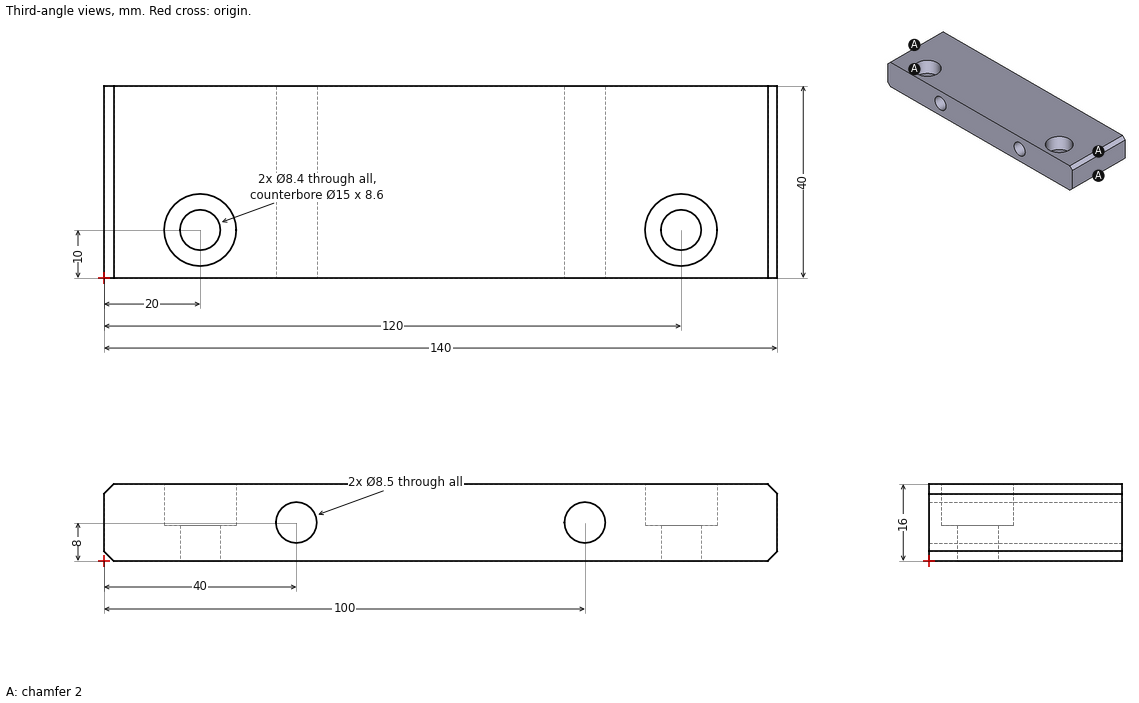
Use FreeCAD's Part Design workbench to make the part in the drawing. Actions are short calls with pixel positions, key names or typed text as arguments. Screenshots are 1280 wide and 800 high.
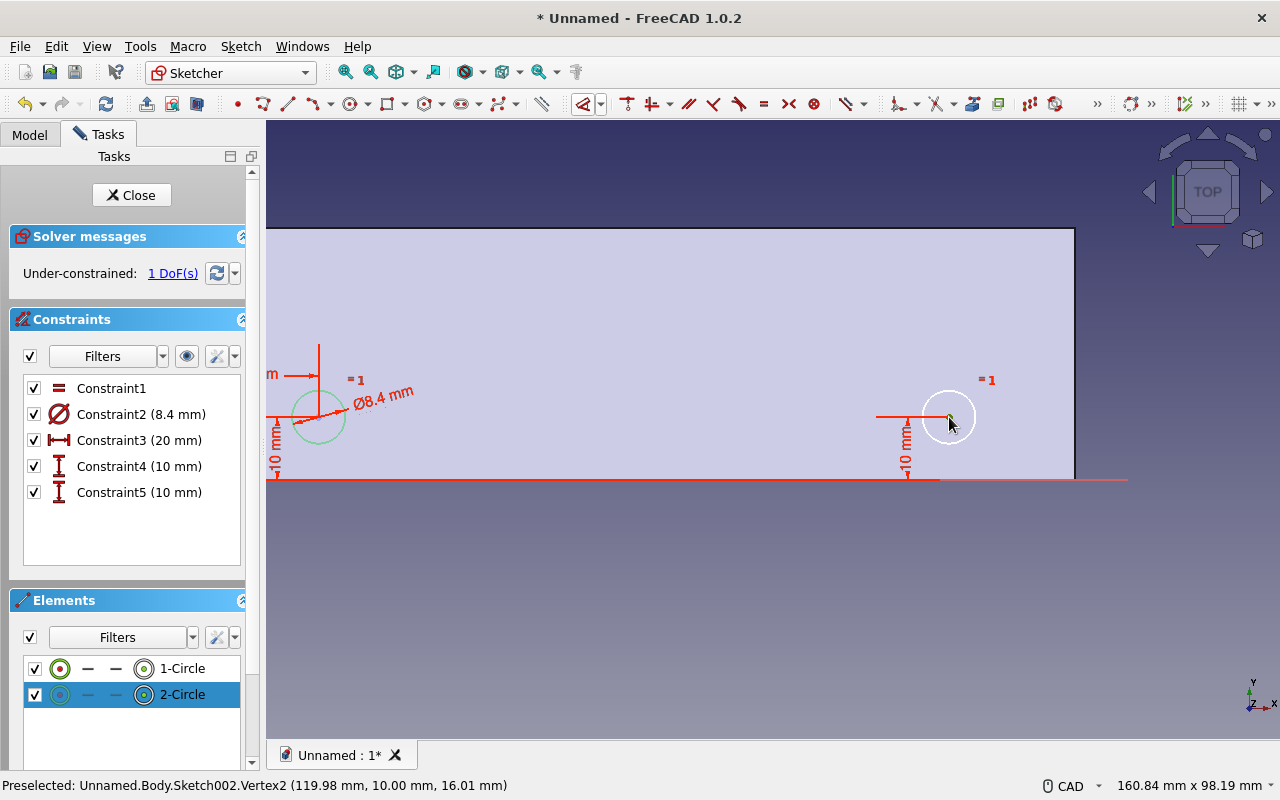
click(600, 104)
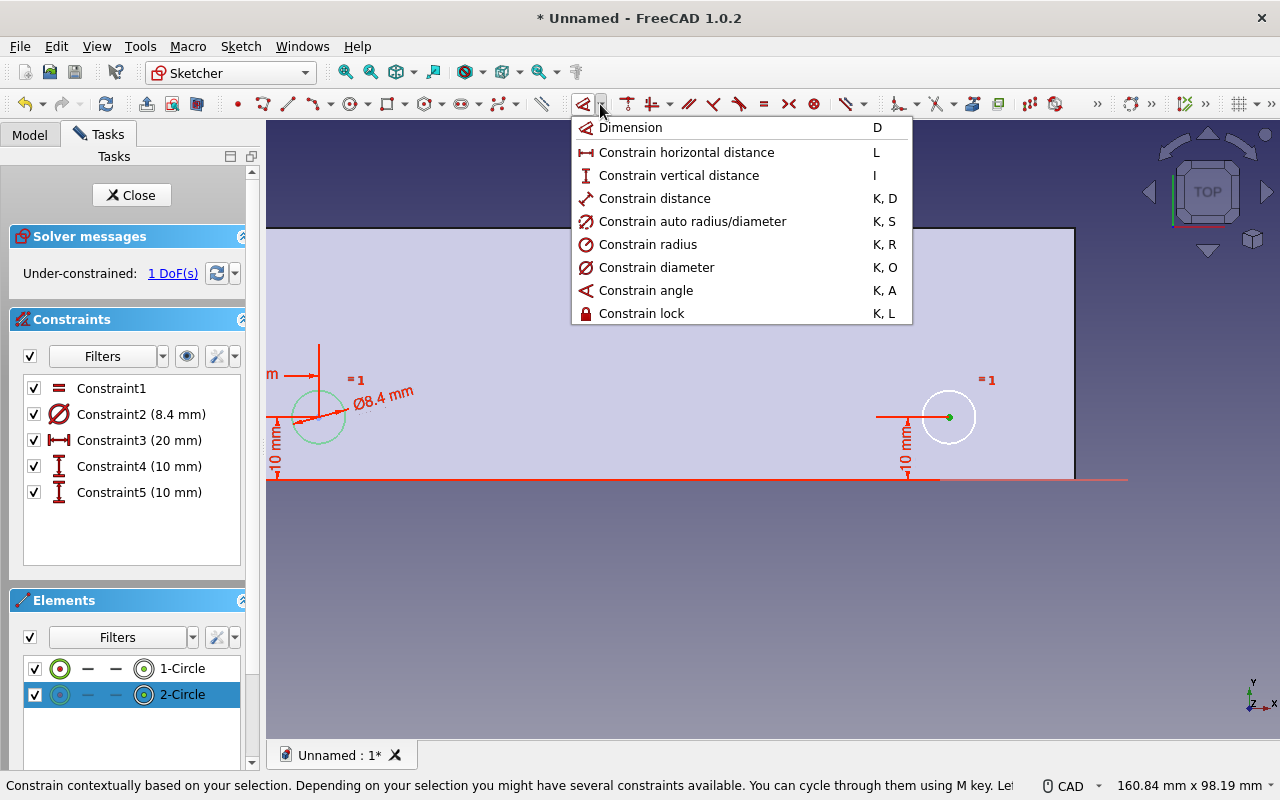
click(742, 152)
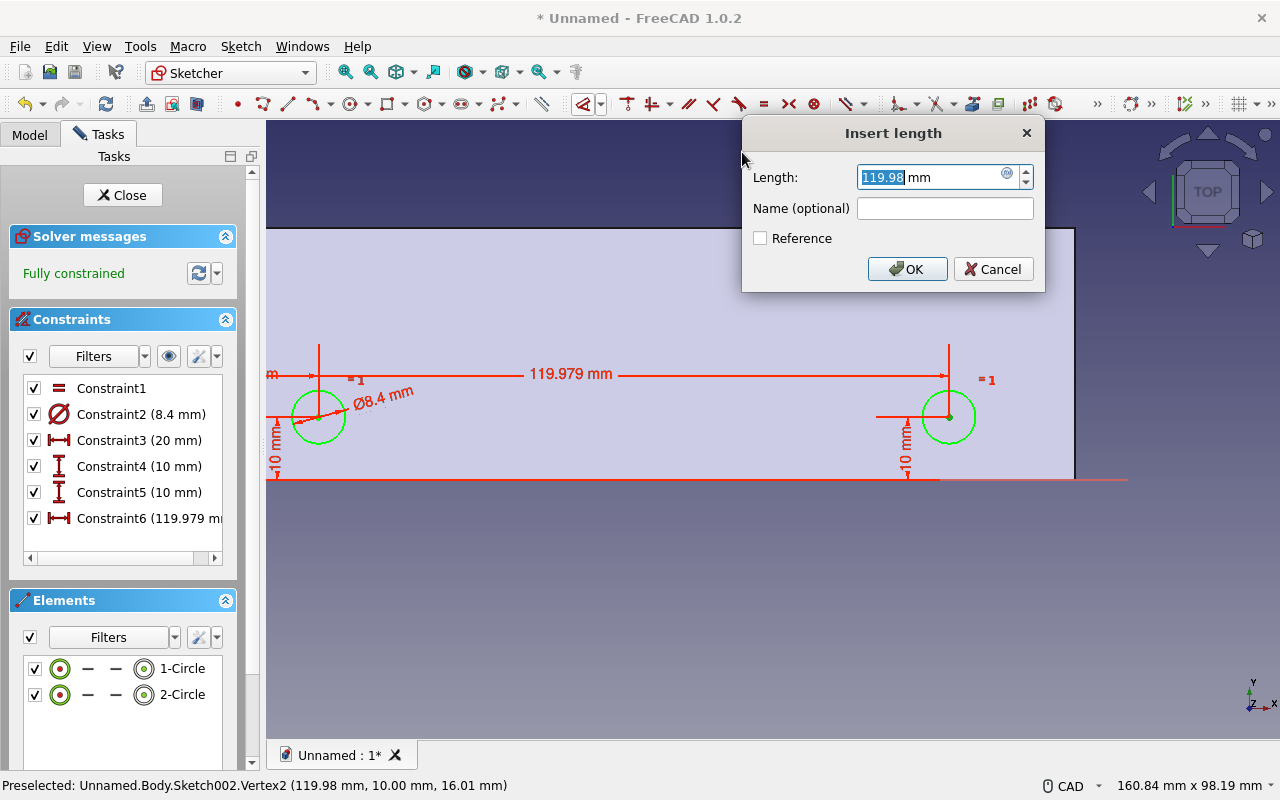
text(120)
key(Return)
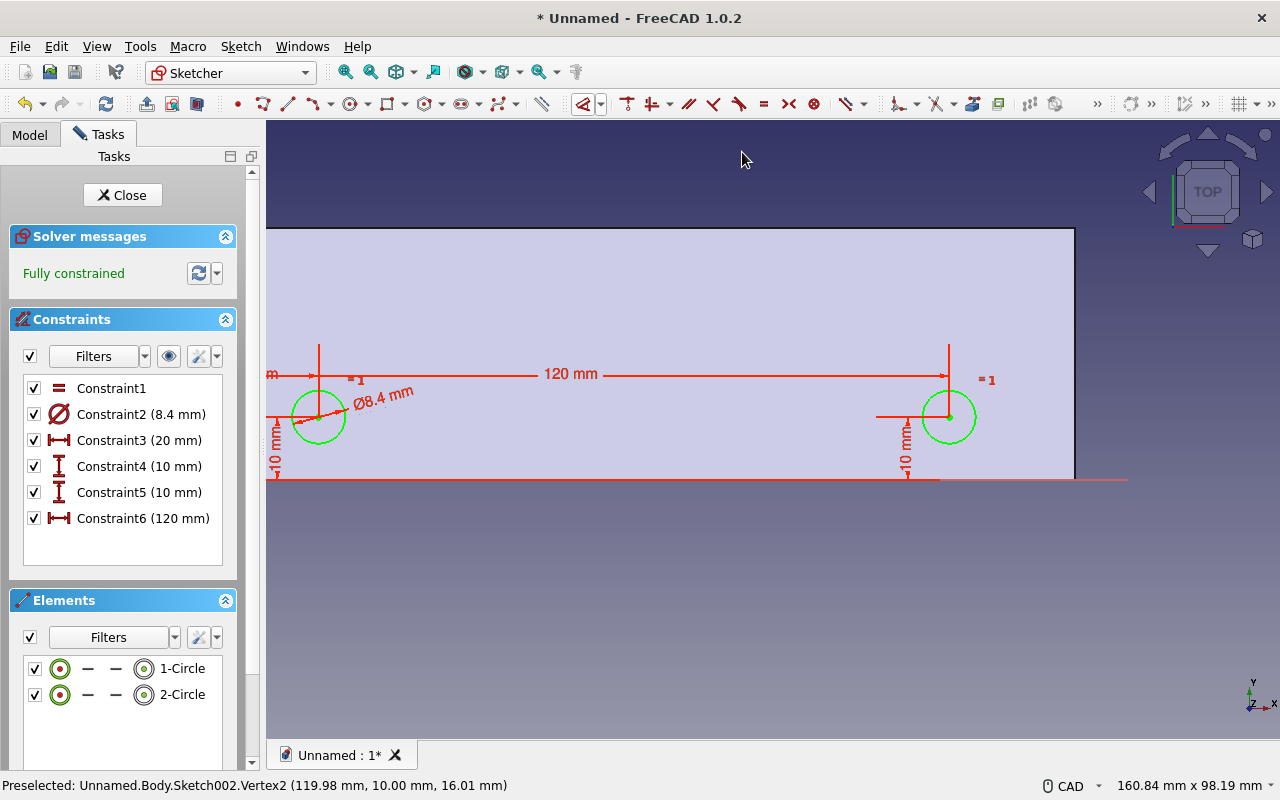
click(123, 195)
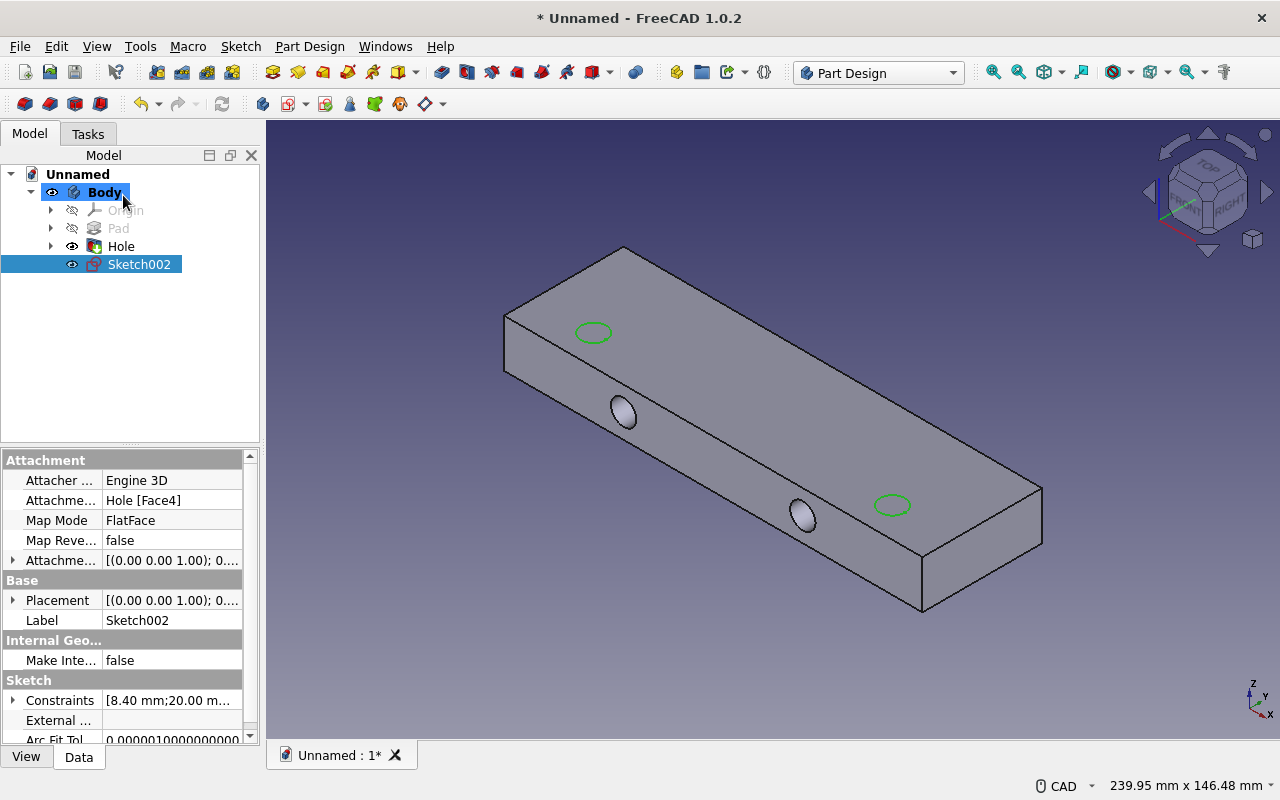
click(467, 72)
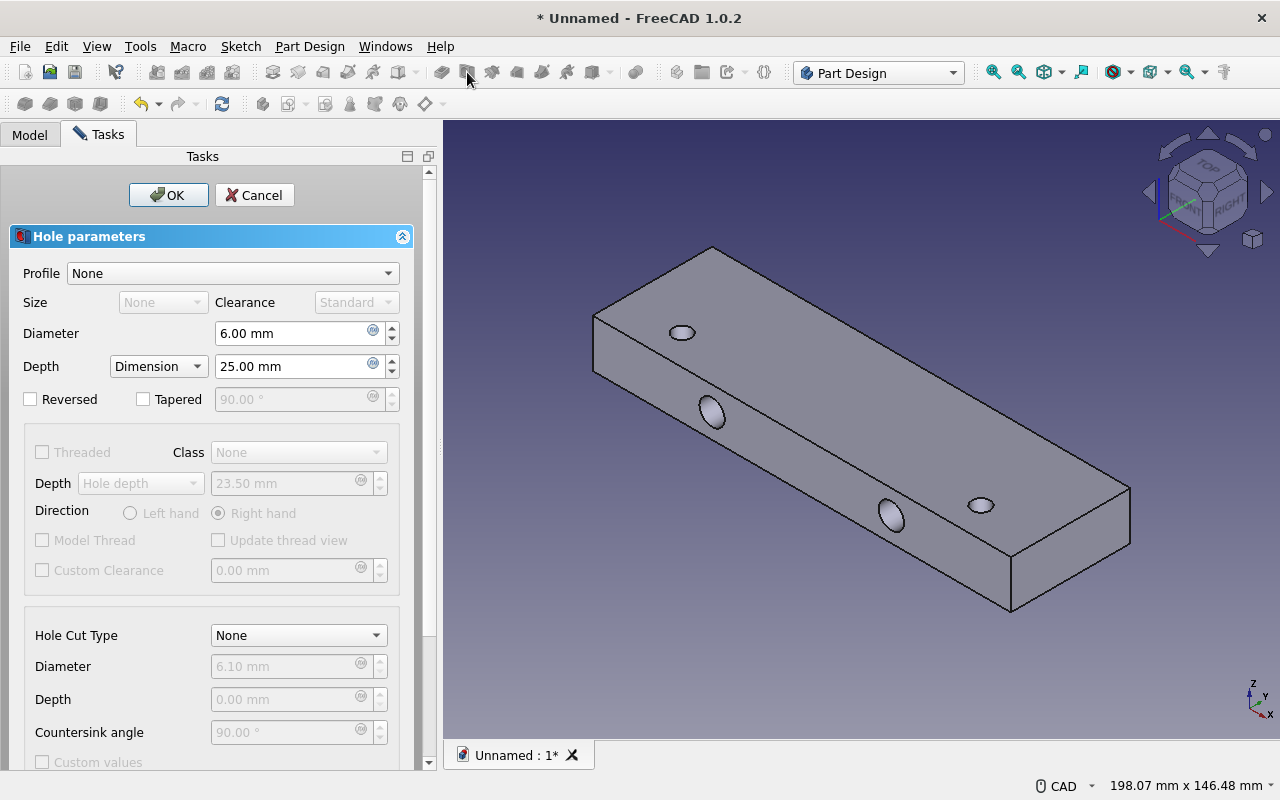
triple_click(300, 334)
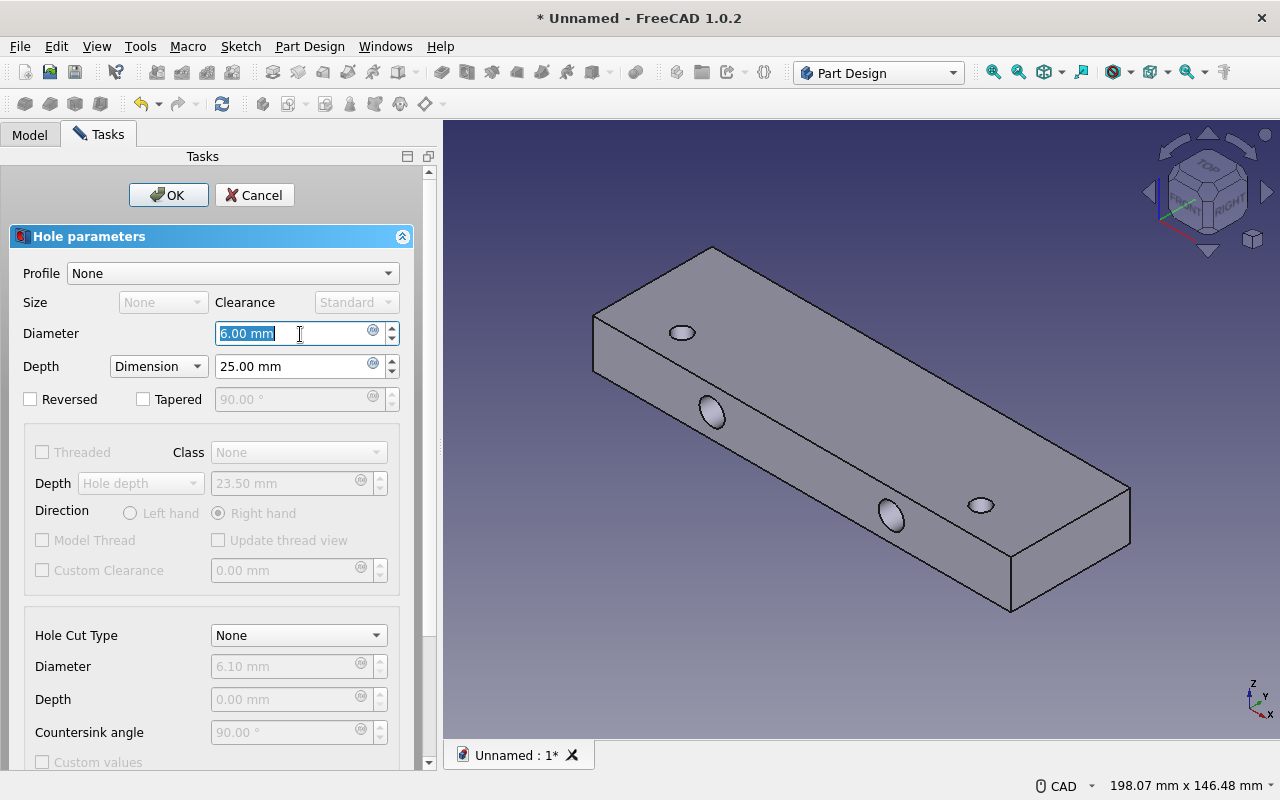
text(8.4)
key(Tab)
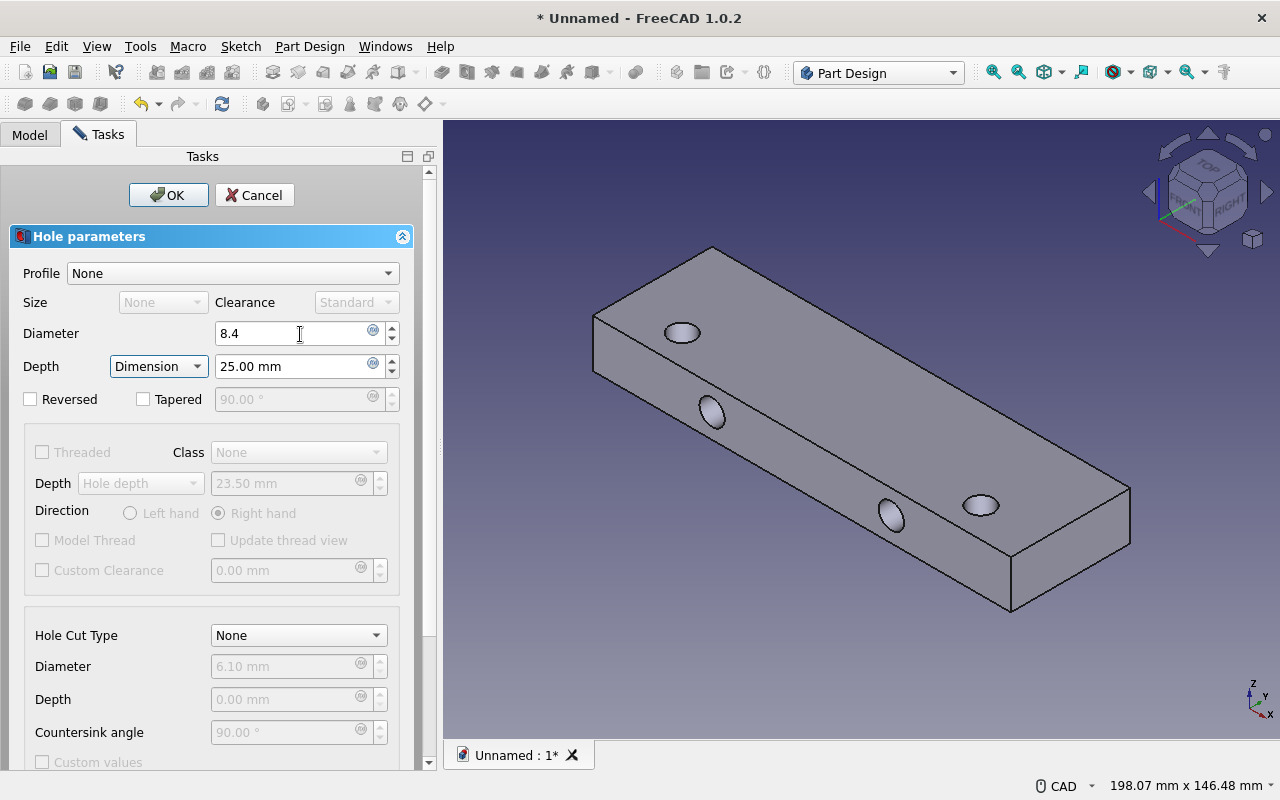
click(160, 366)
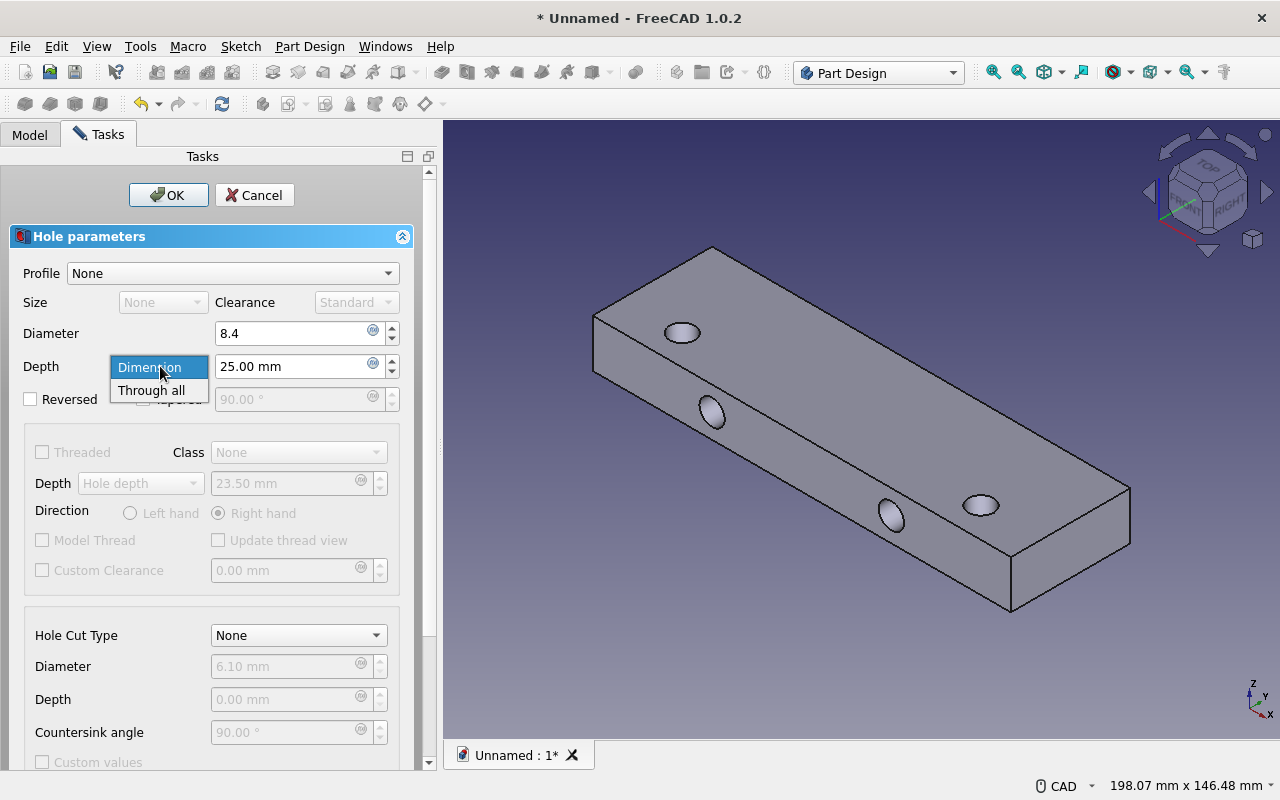
click(158, 390)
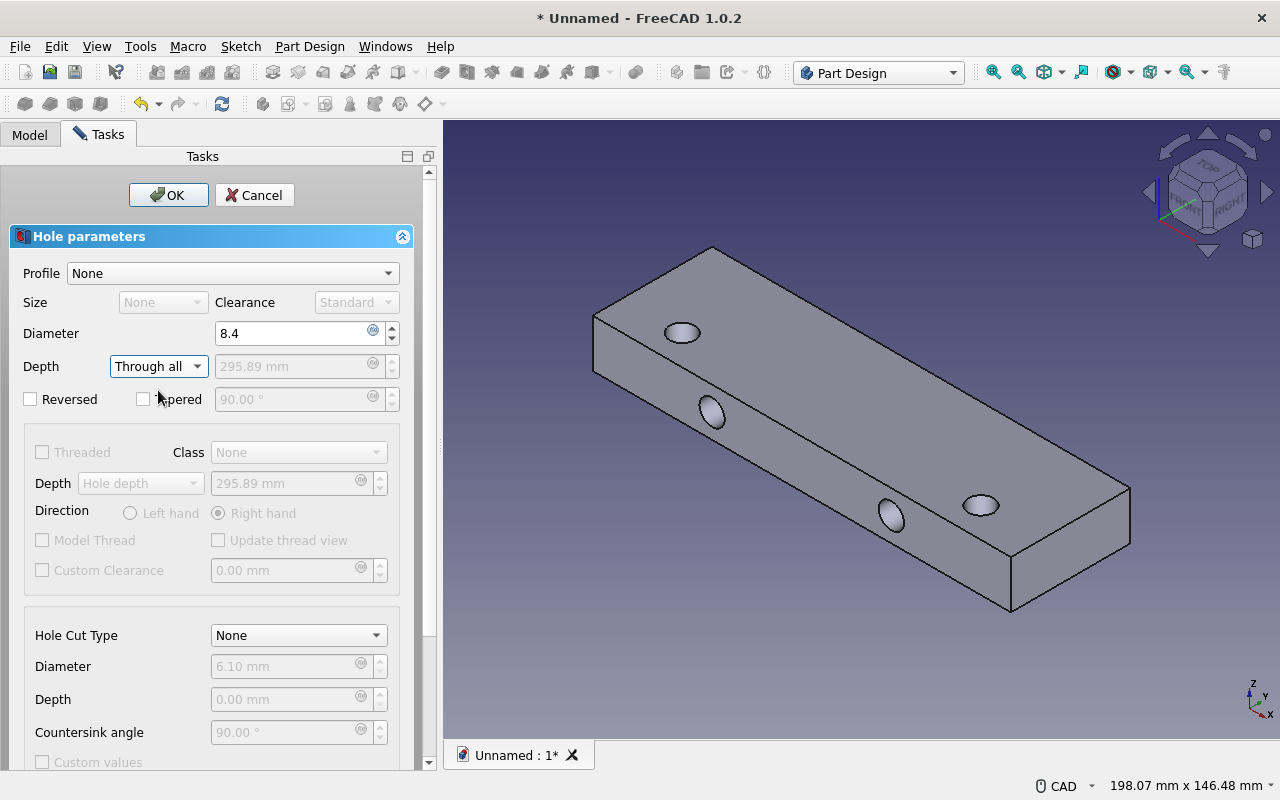
click(300, 636)